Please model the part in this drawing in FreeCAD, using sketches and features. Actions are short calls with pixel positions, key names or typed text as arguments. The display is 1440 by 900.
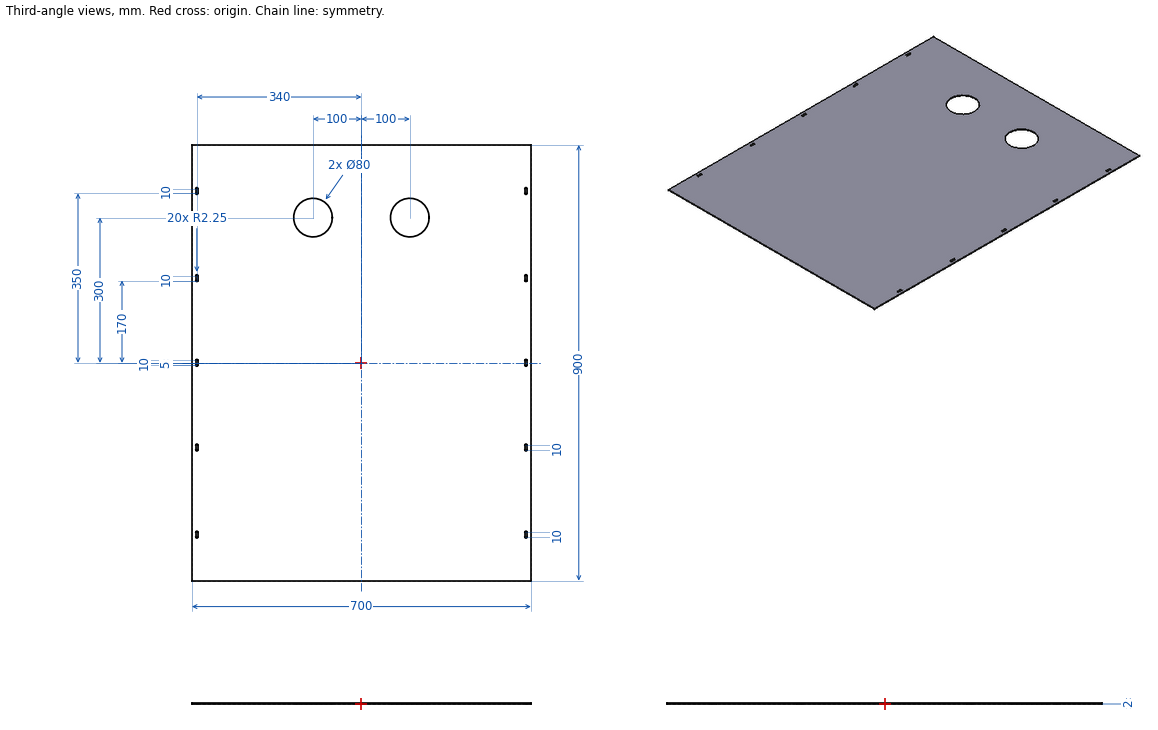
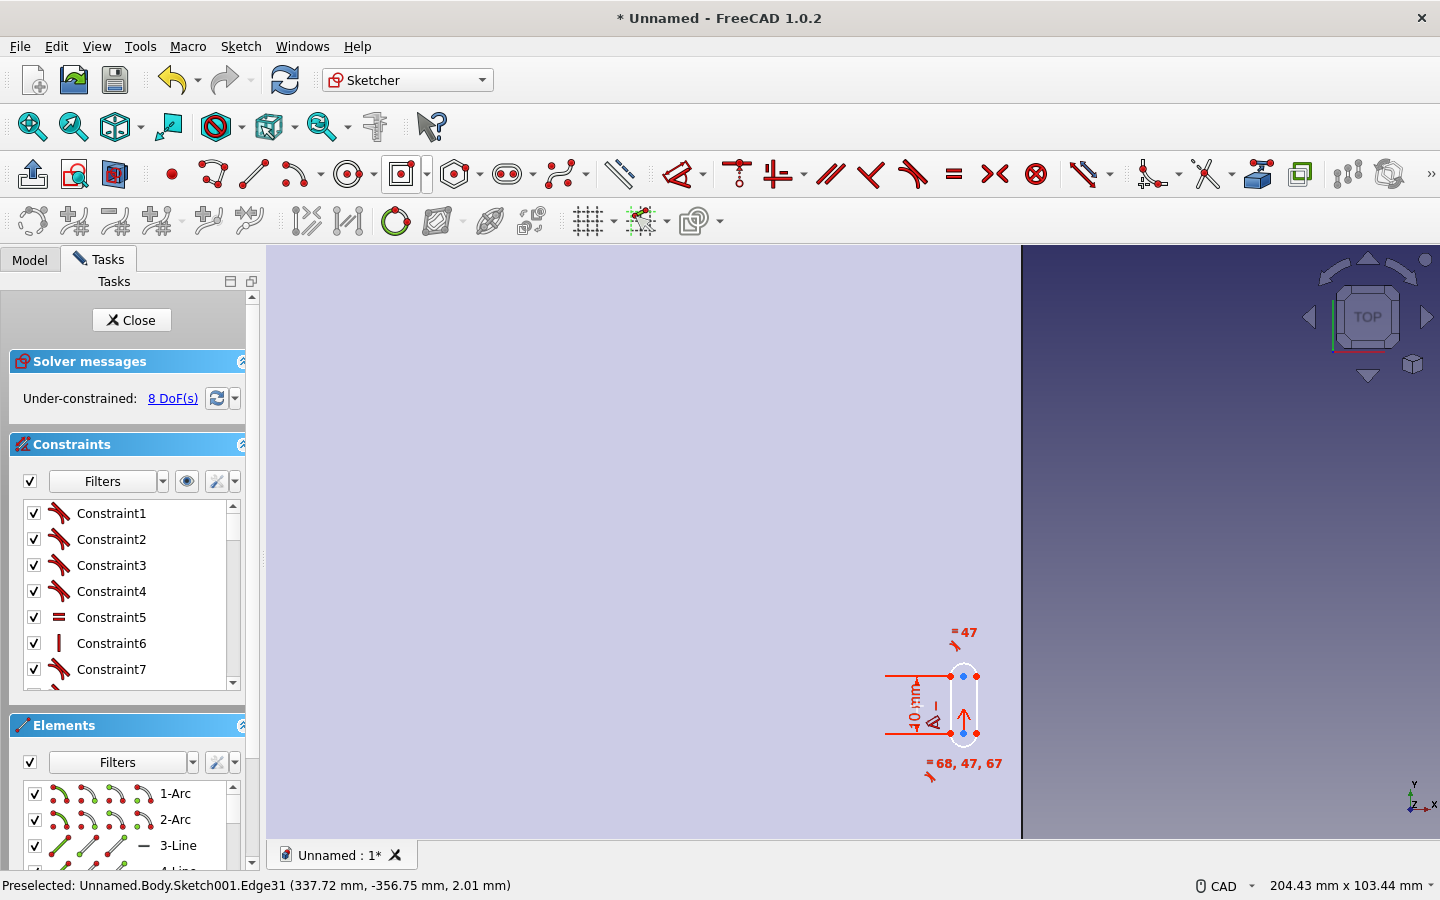
scroll(961, 729, down, 12)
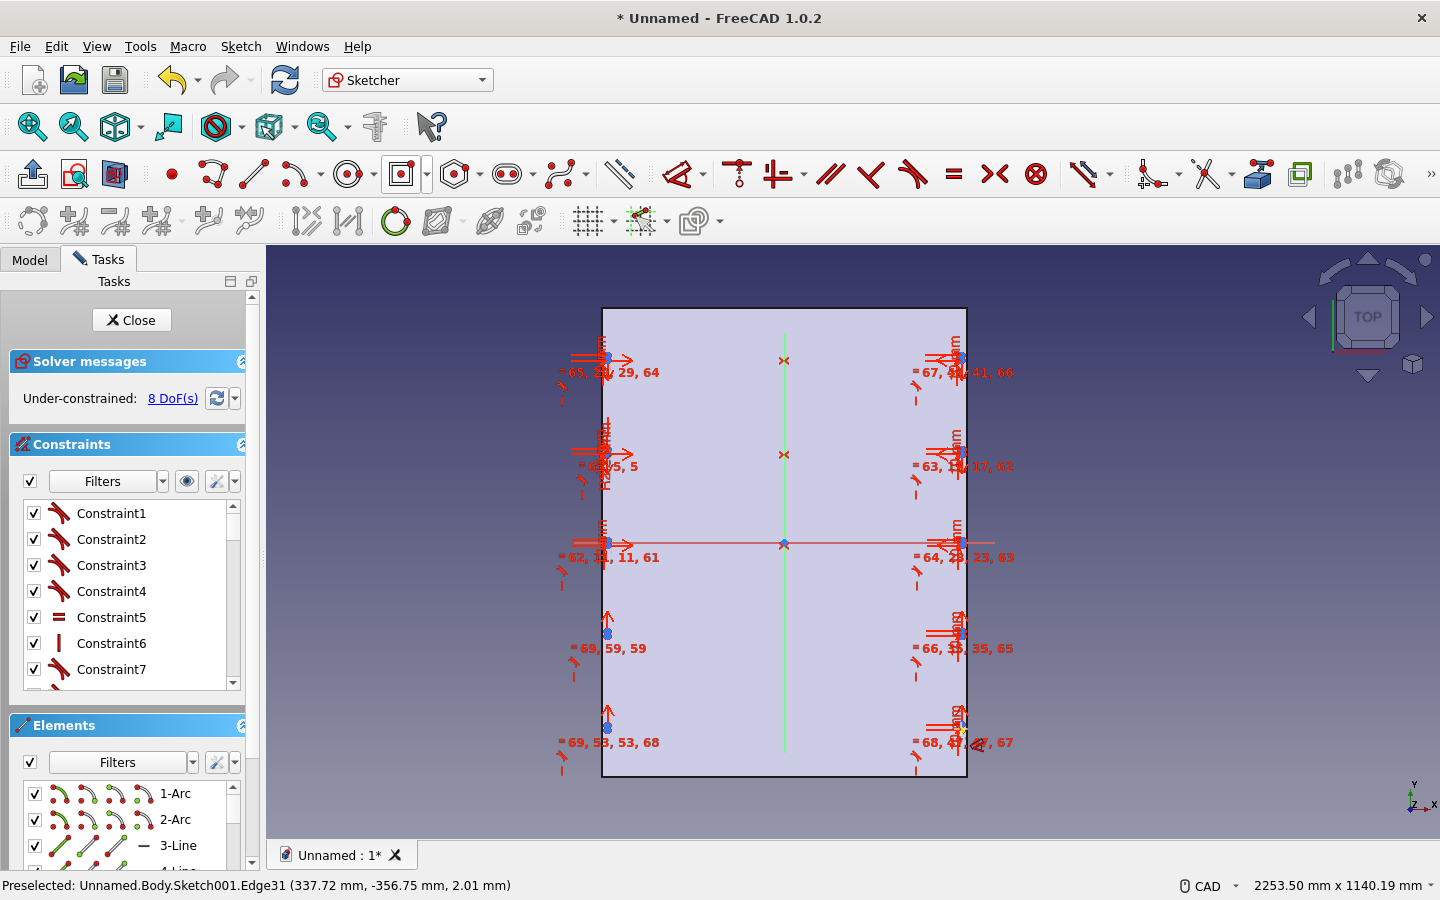
scroll(606, 729, up, 12)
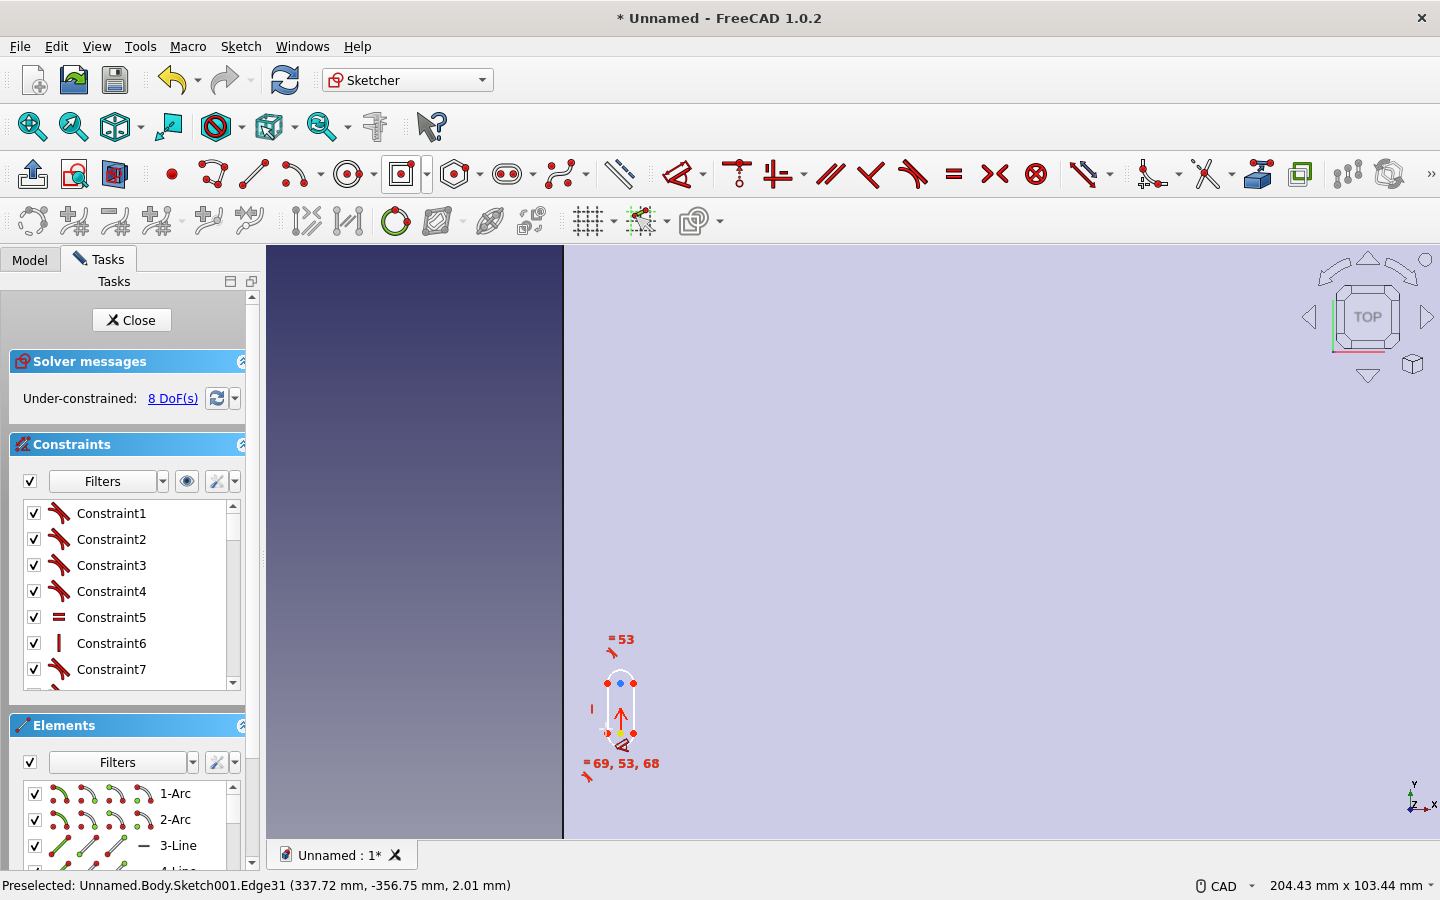
click(608, 719)
click(574, 709)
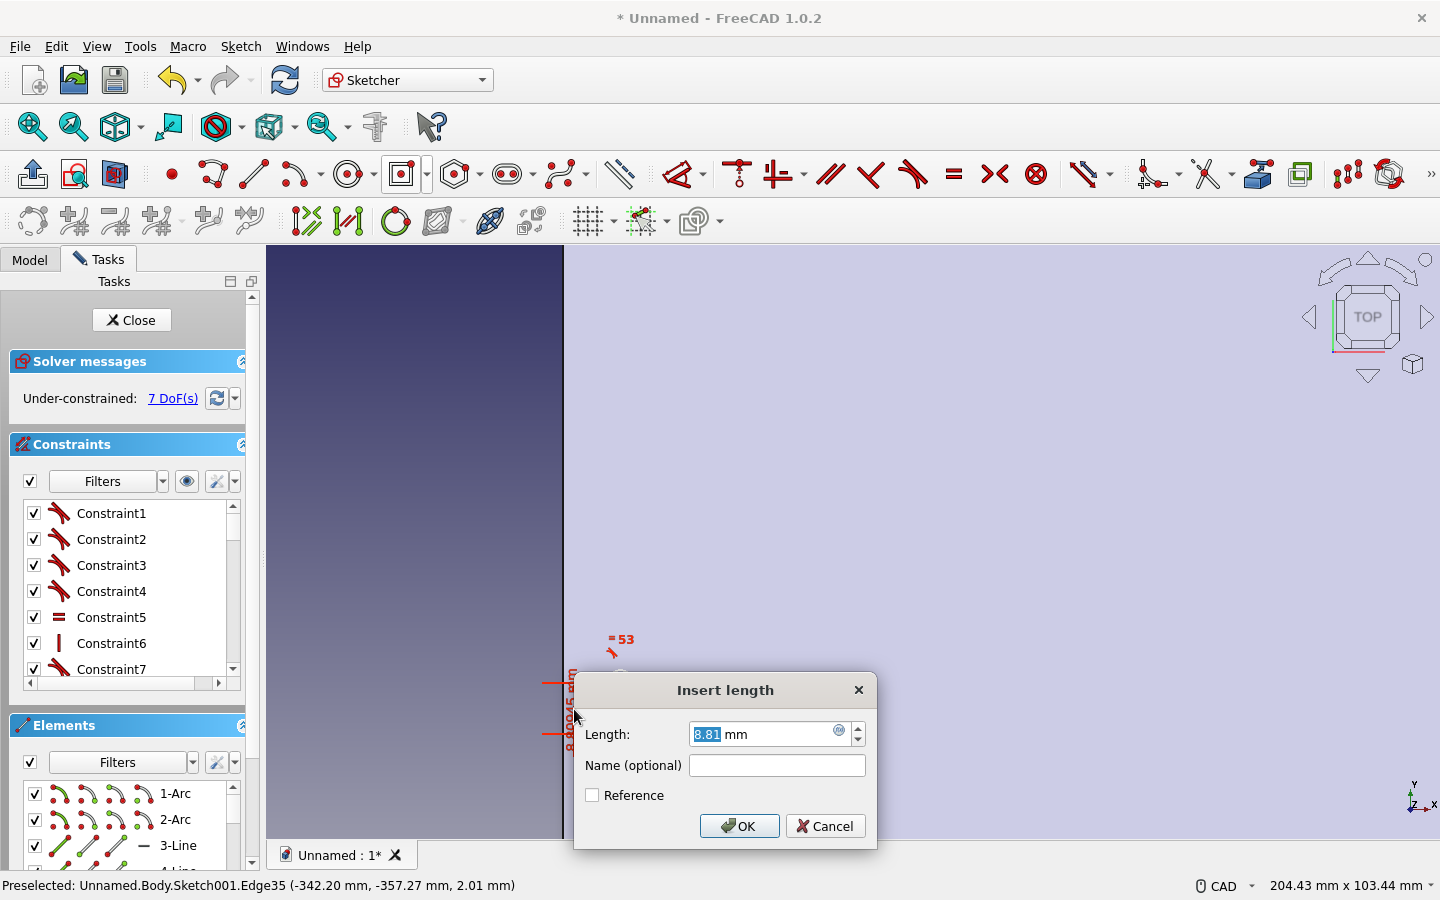
text(10)
key(Return)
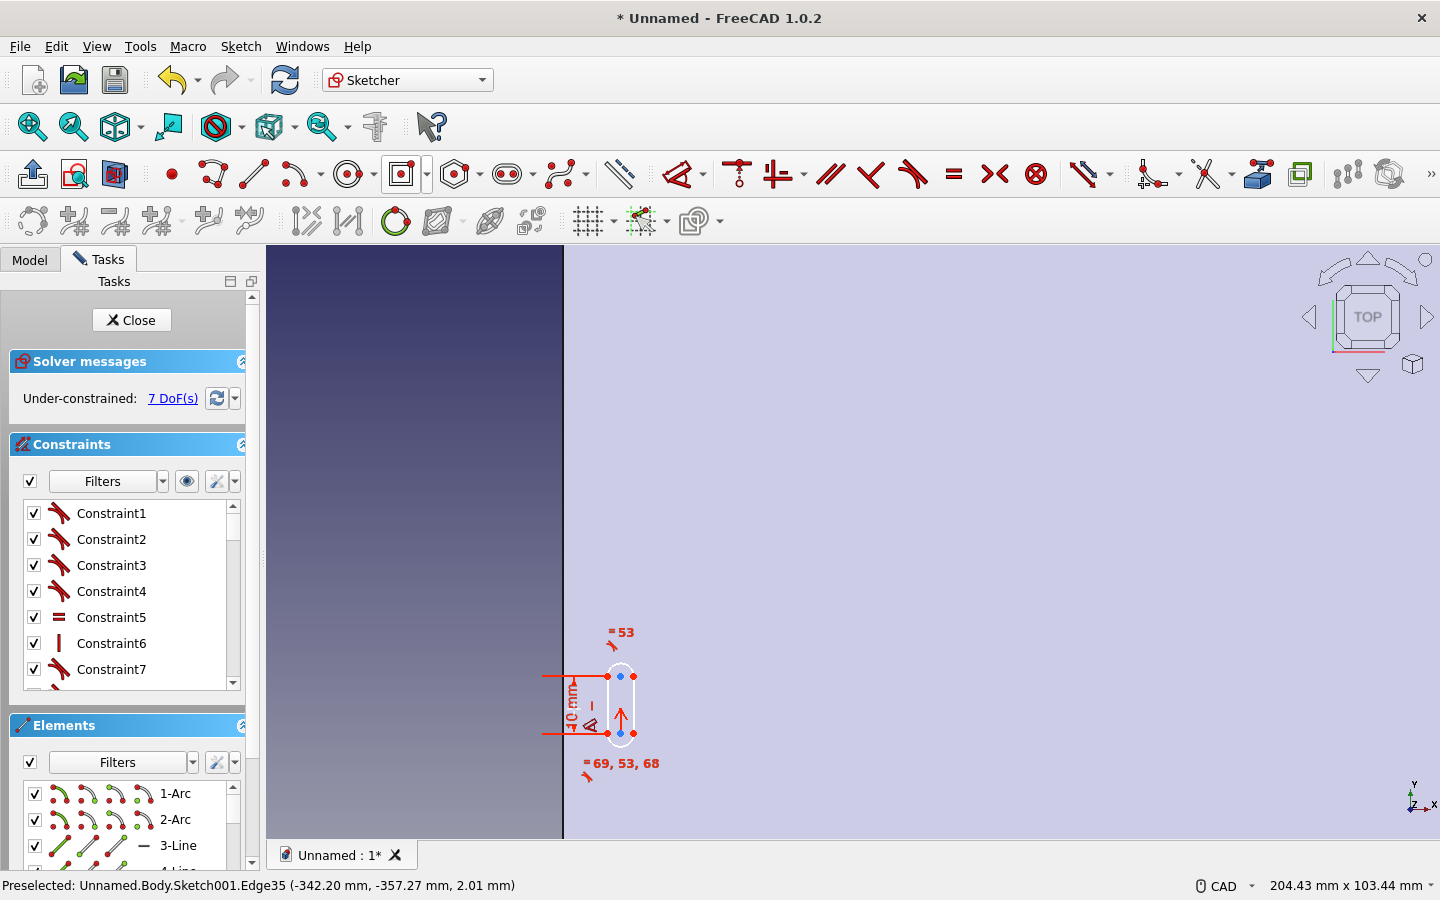
scroll(606, 729, down, 12)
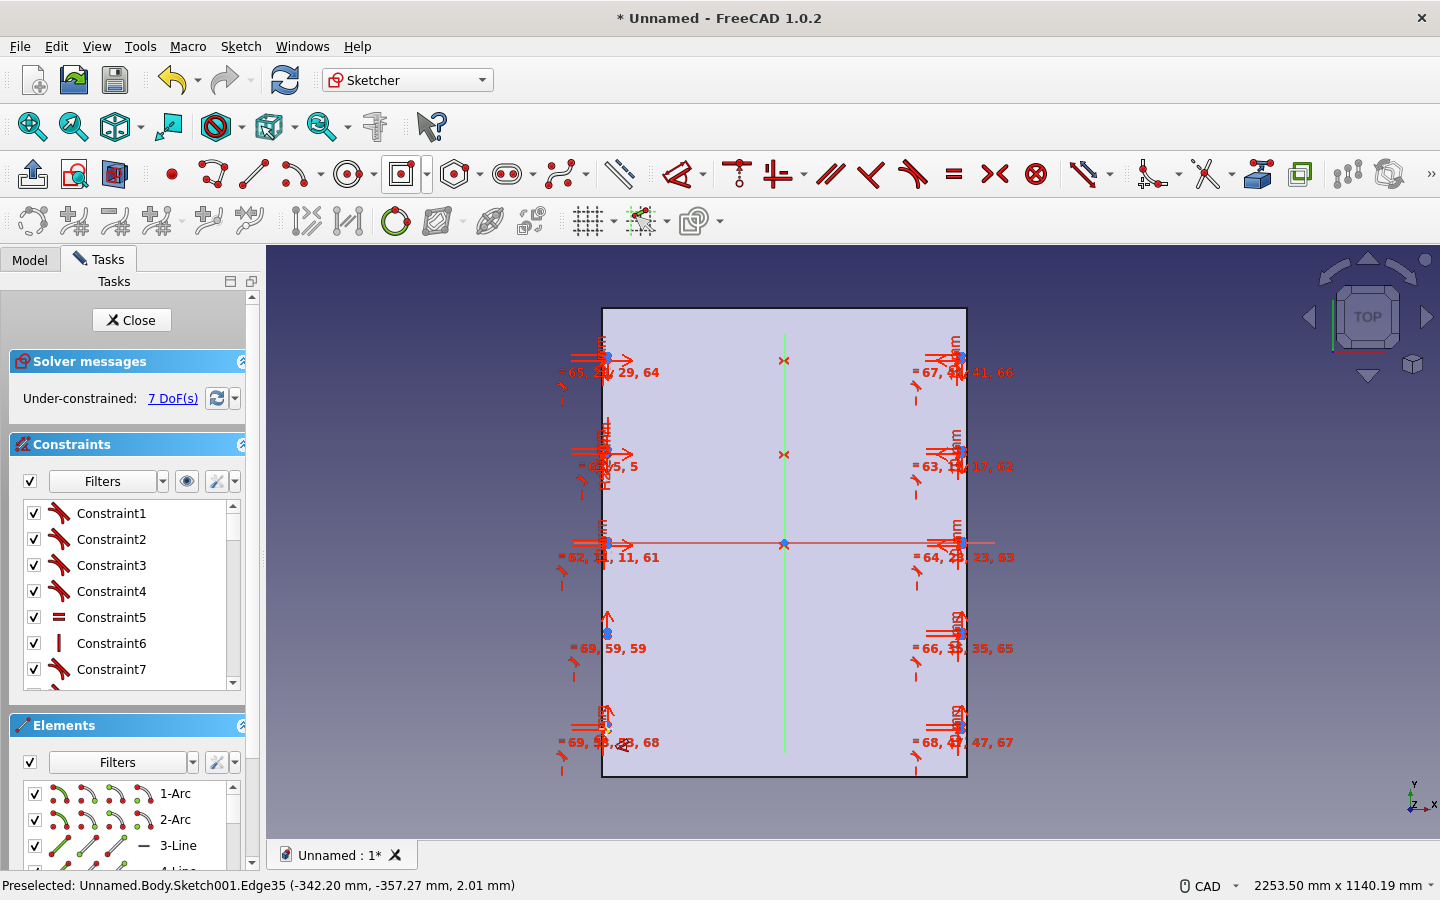
scroll(606, 635, up, 12)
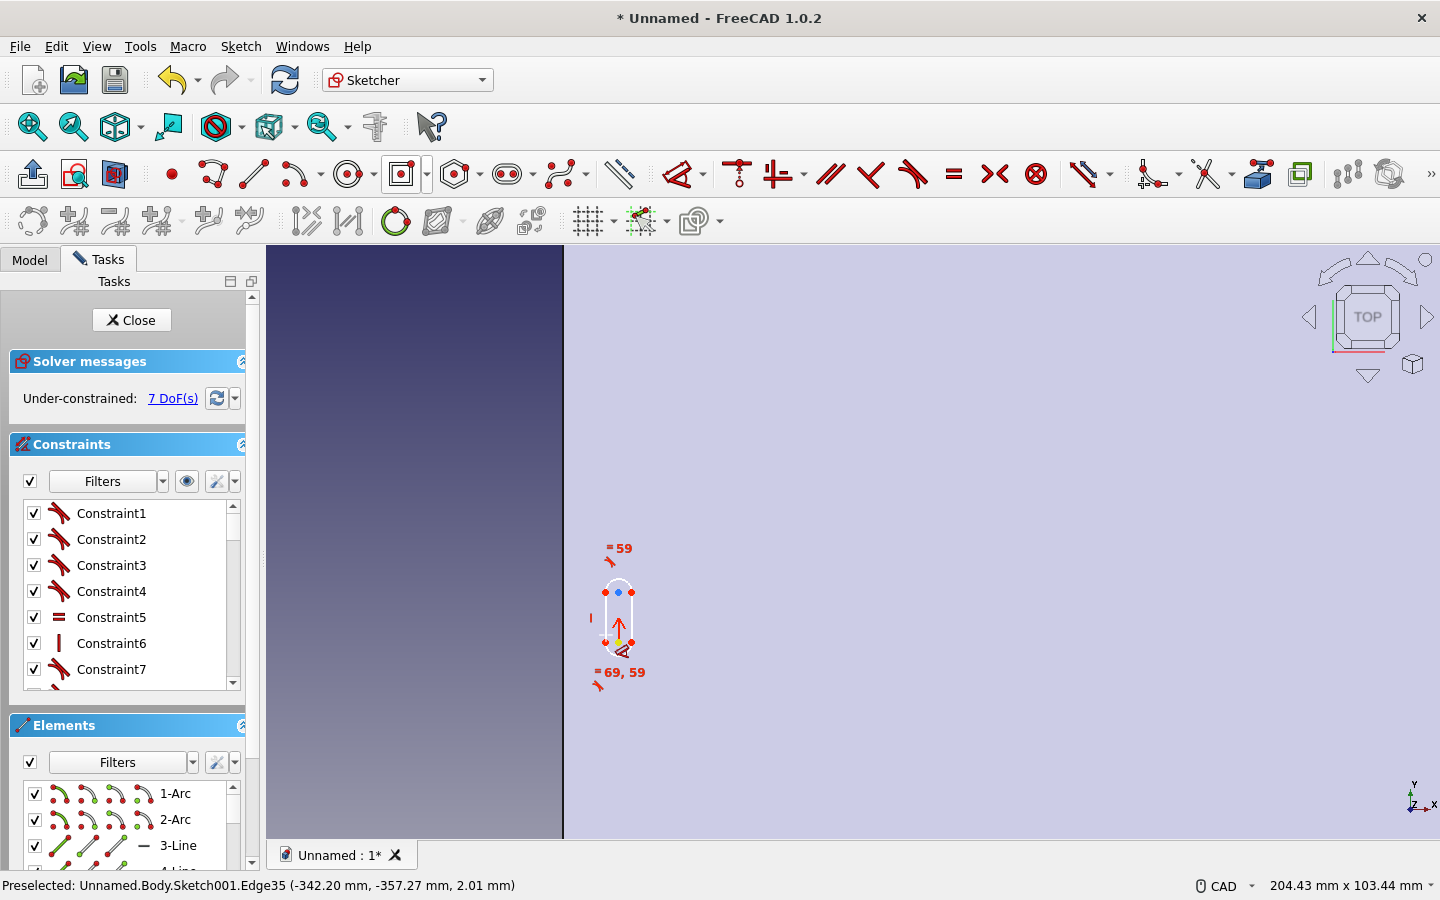
click(606, 628)
click(572, 617)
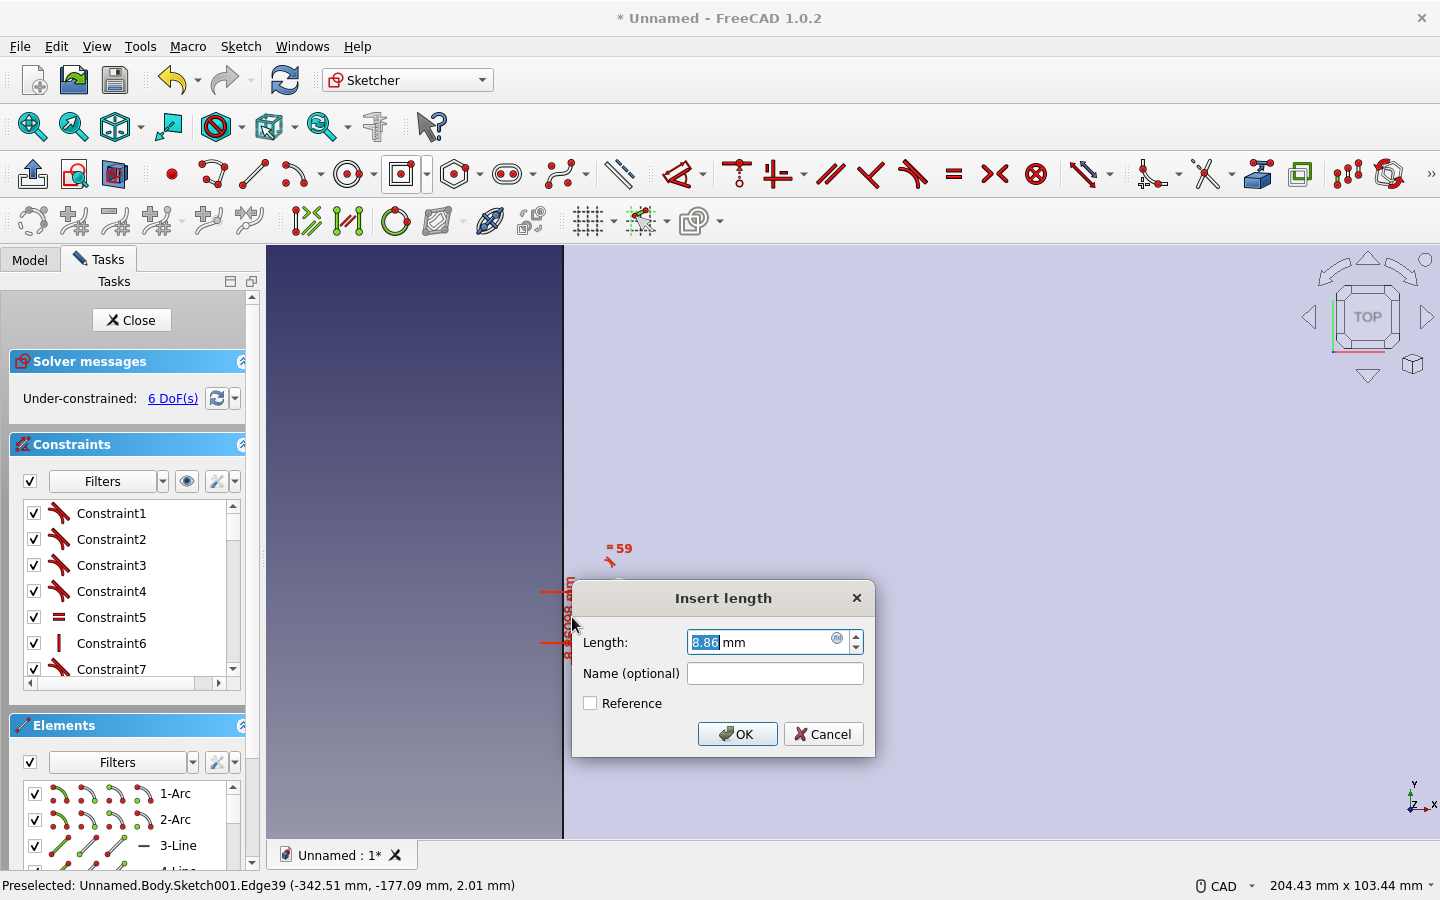
text(10)
key(Return)